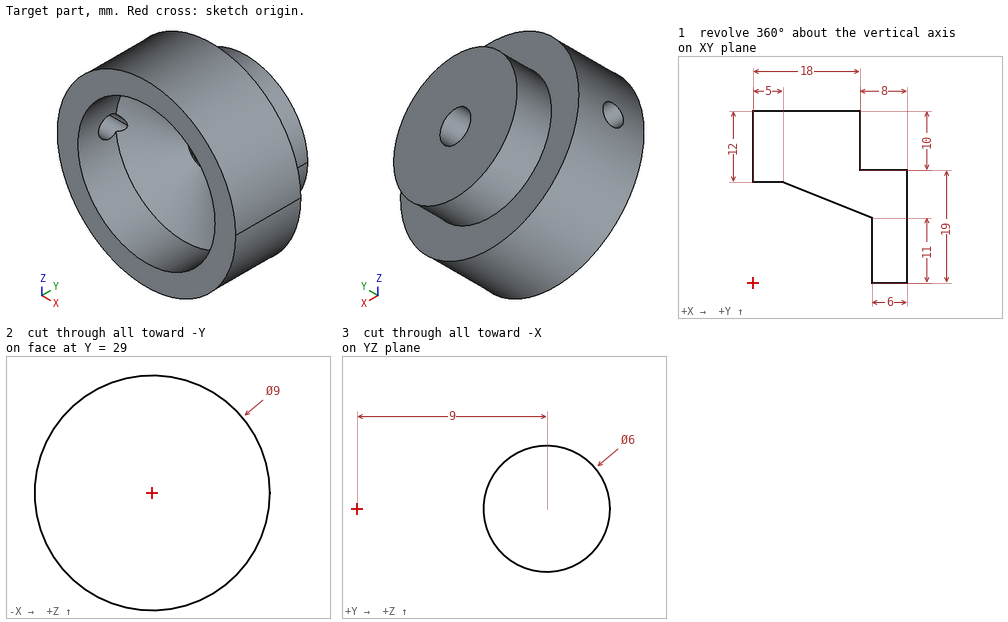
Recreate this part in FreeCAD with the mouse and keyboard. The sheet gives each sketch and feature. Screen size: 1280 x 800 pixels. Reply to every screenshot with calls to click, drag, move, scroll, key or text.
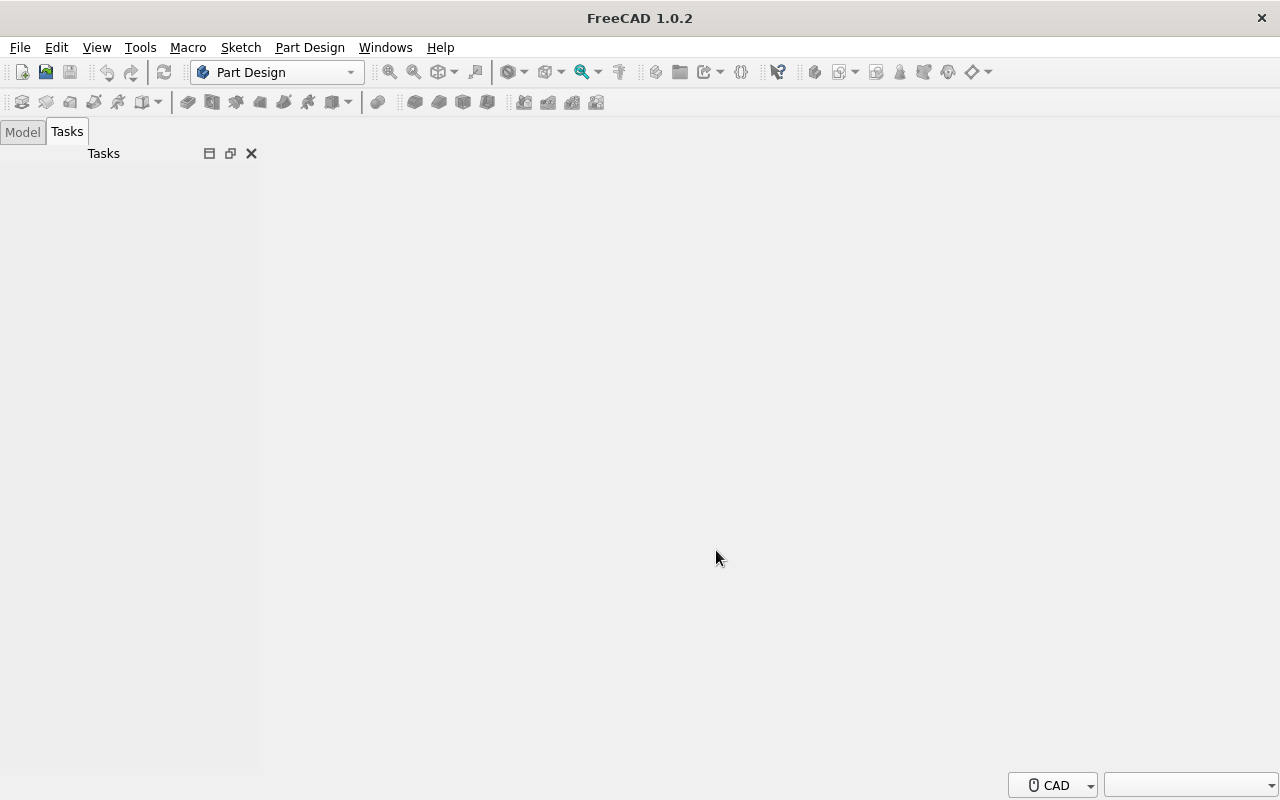
click(22, 72)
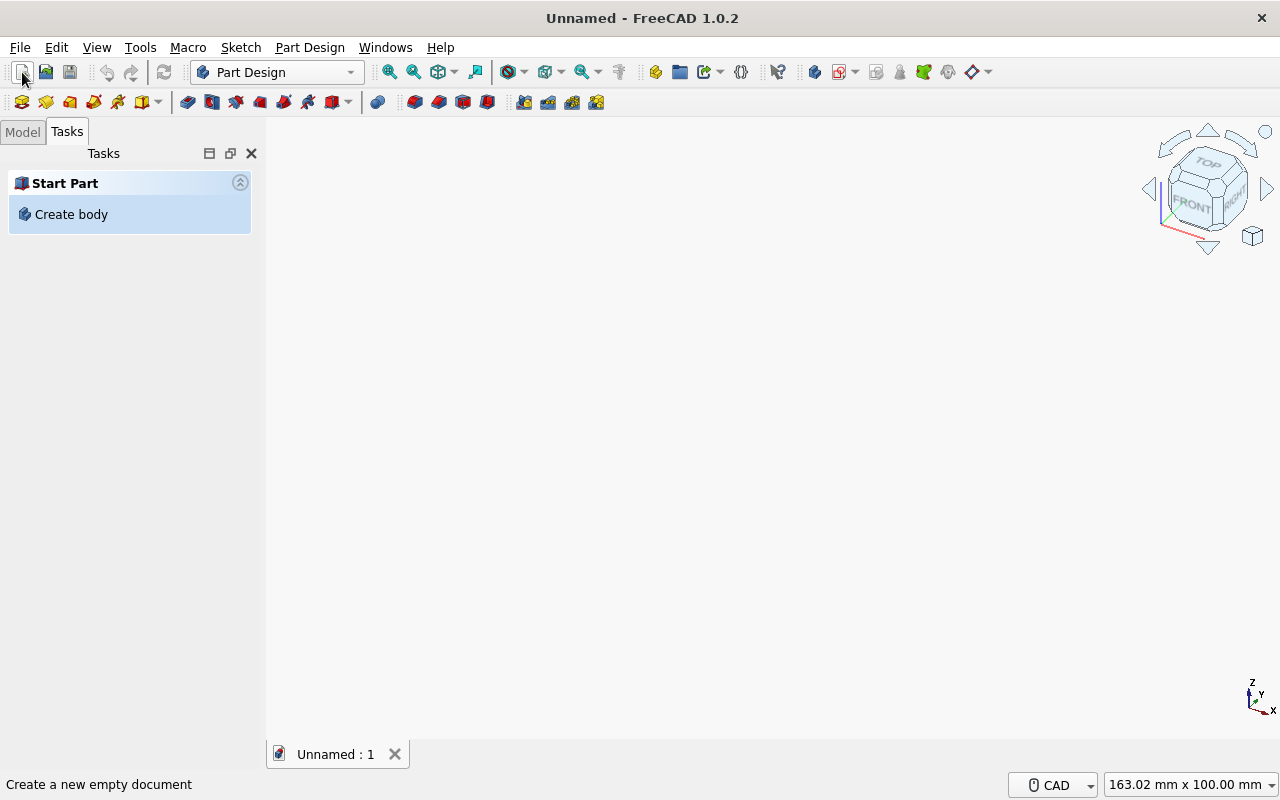
click(840, 72)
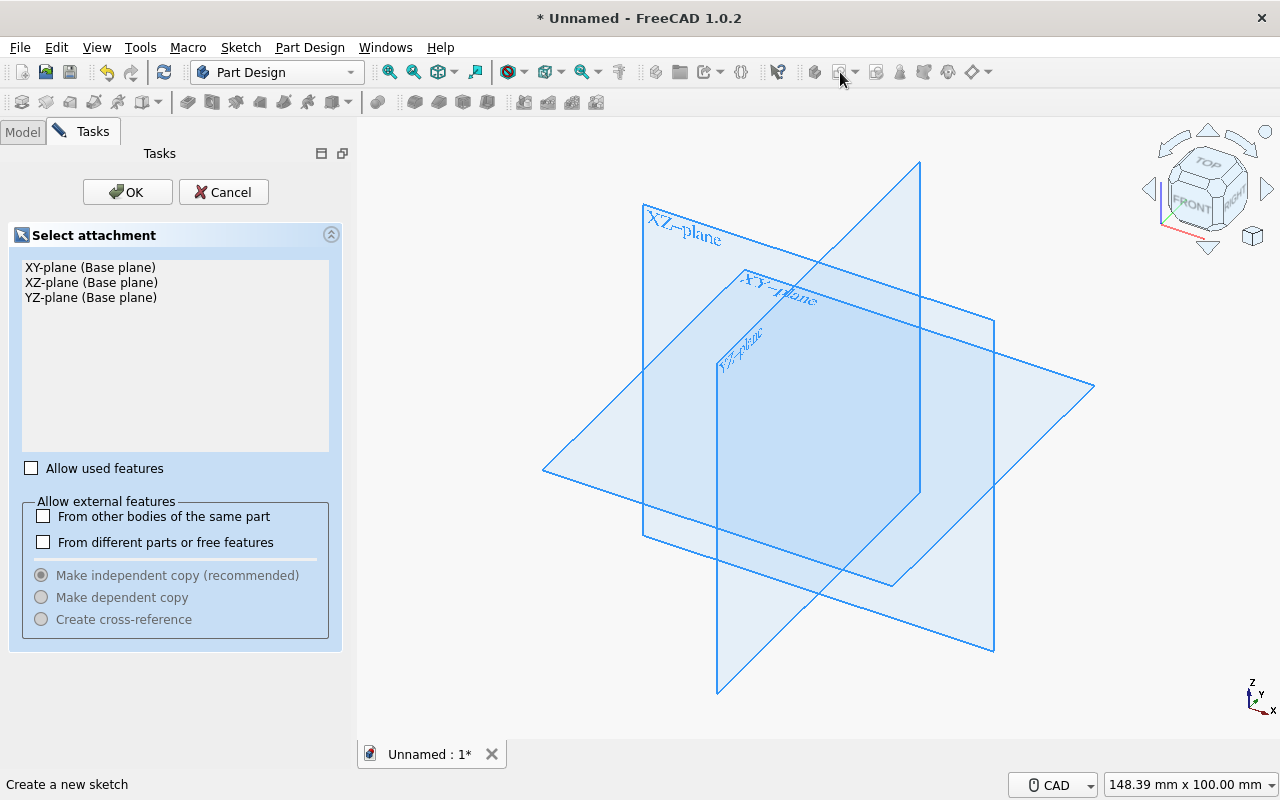
click(82, 268)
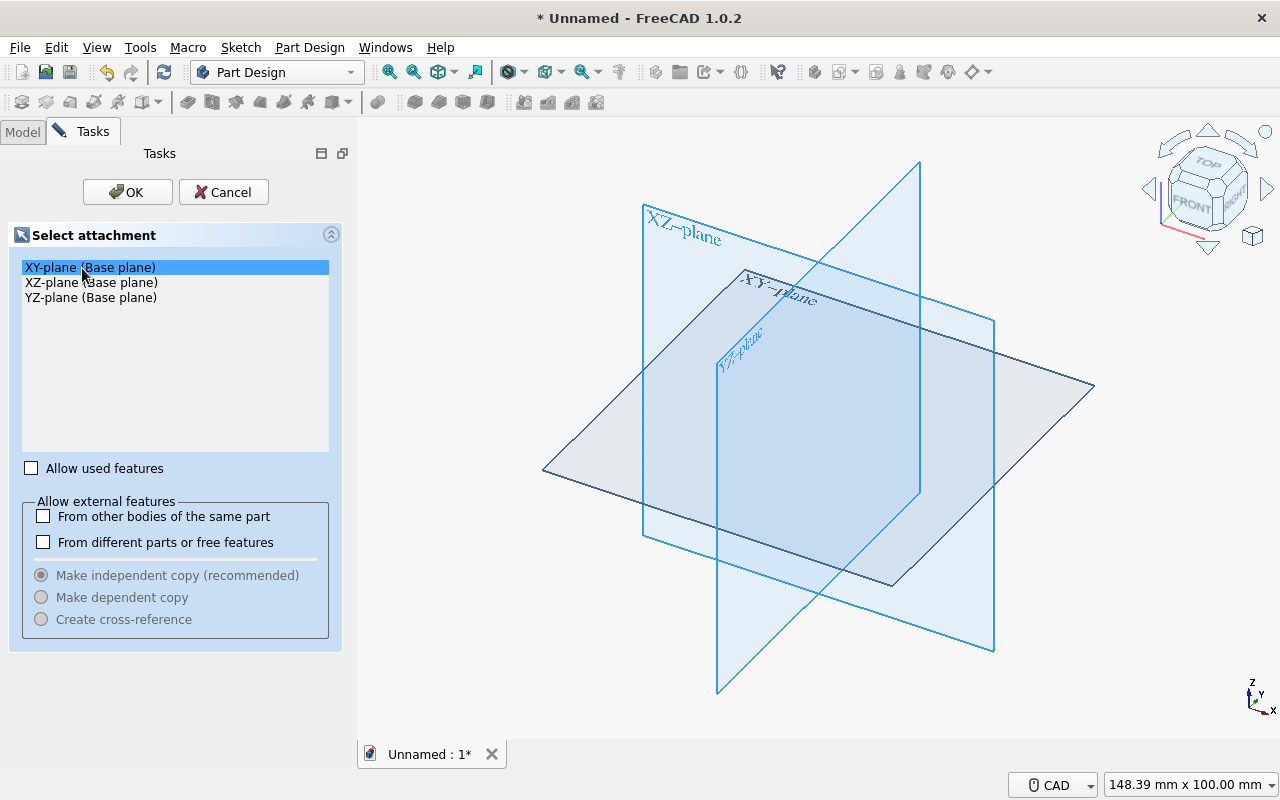
click(128, 192)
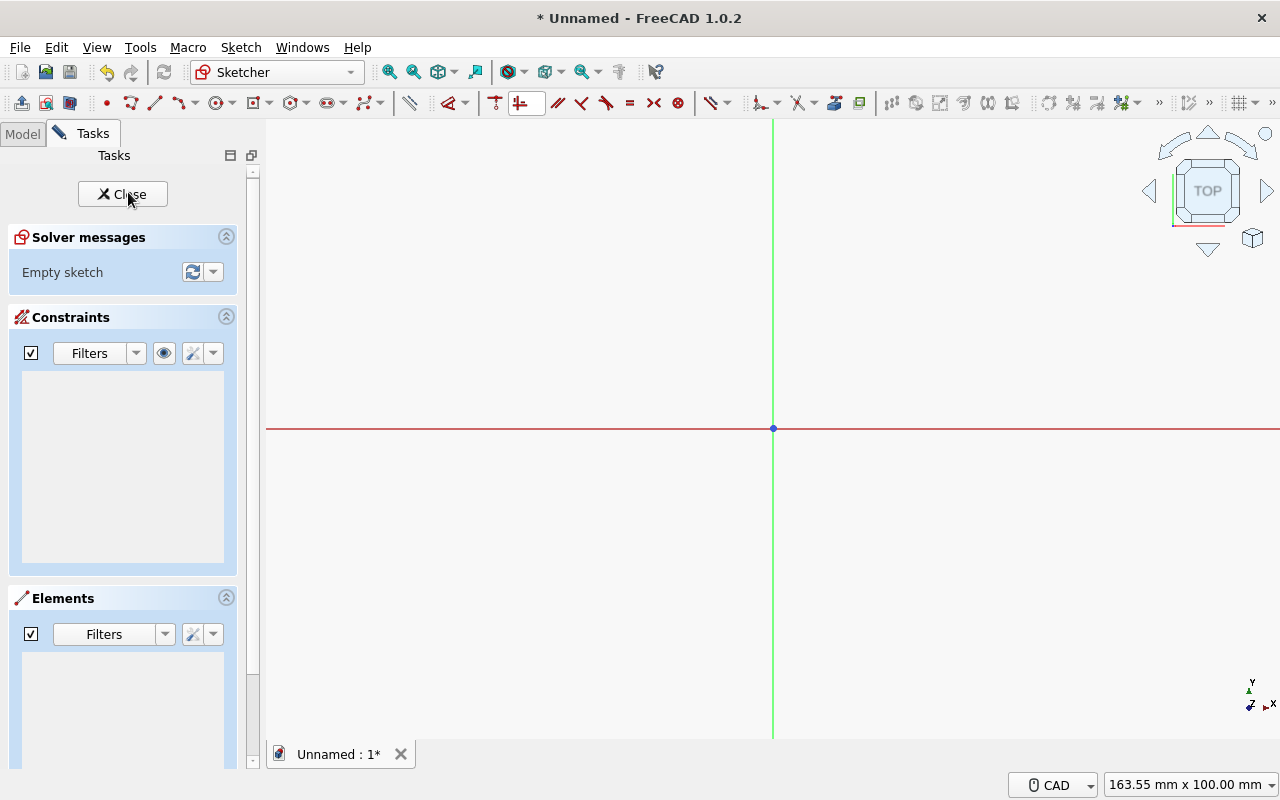
scroll(975, 266, up, 4)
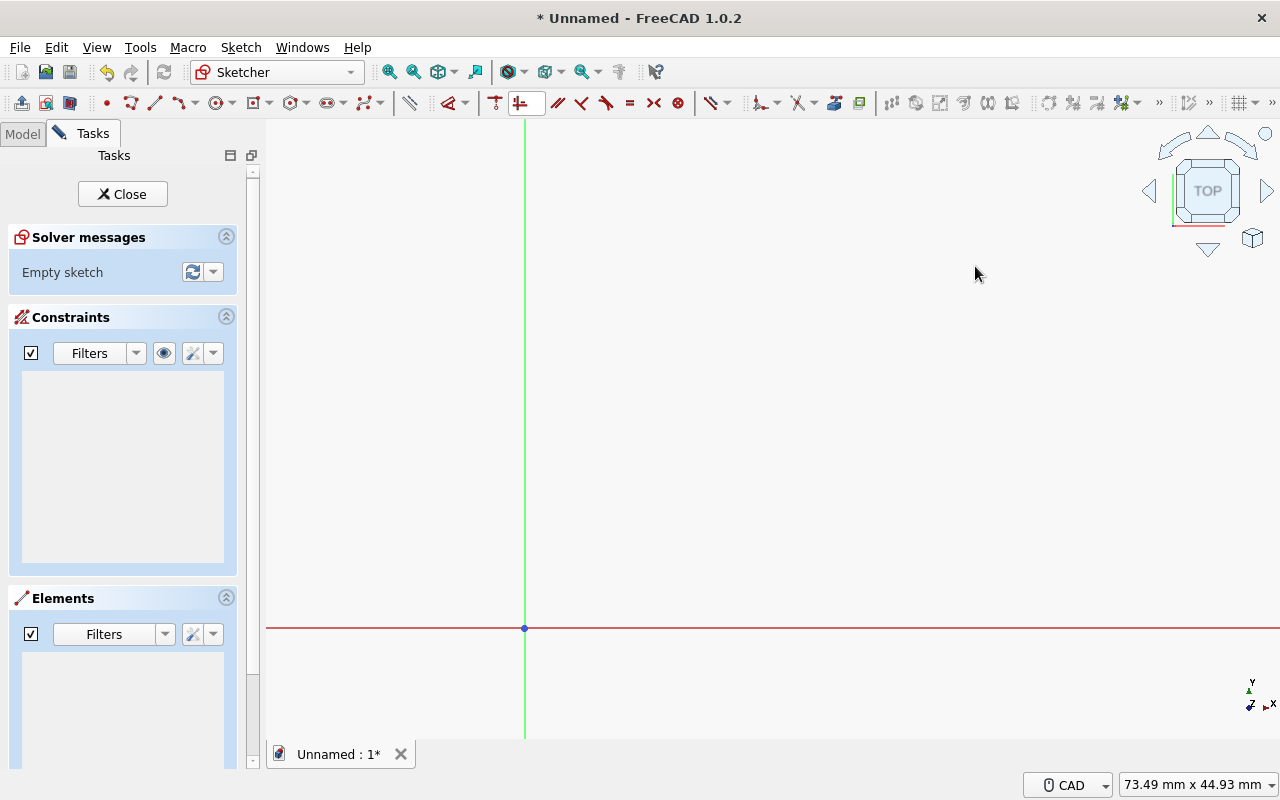
click(132, 104)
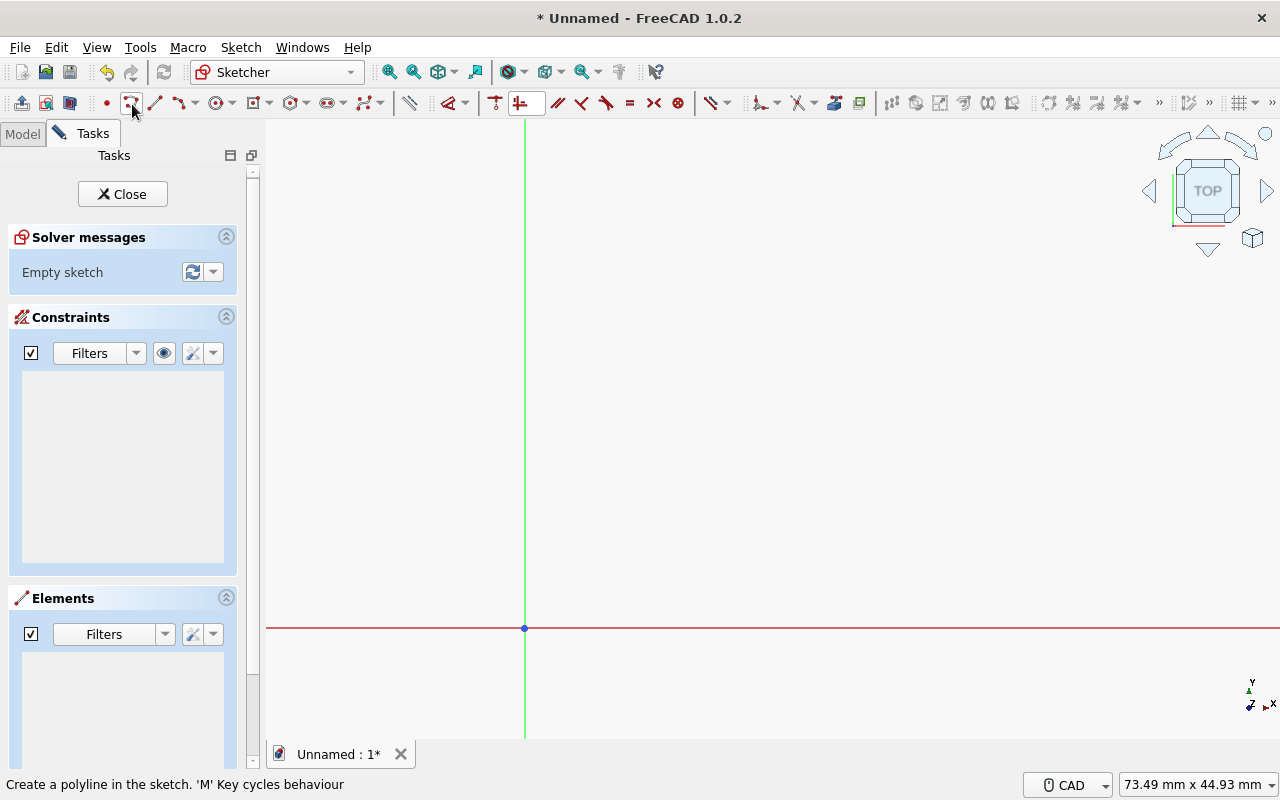
click(525, 394)
click(594, 394)
click(801, 477)
click(801, 628)
click(883, 619)
click(883, 366)
click(773, 366)
click(773, 228)
click(534, 228)
click(525, 395)
key(Escape)
key(Escape)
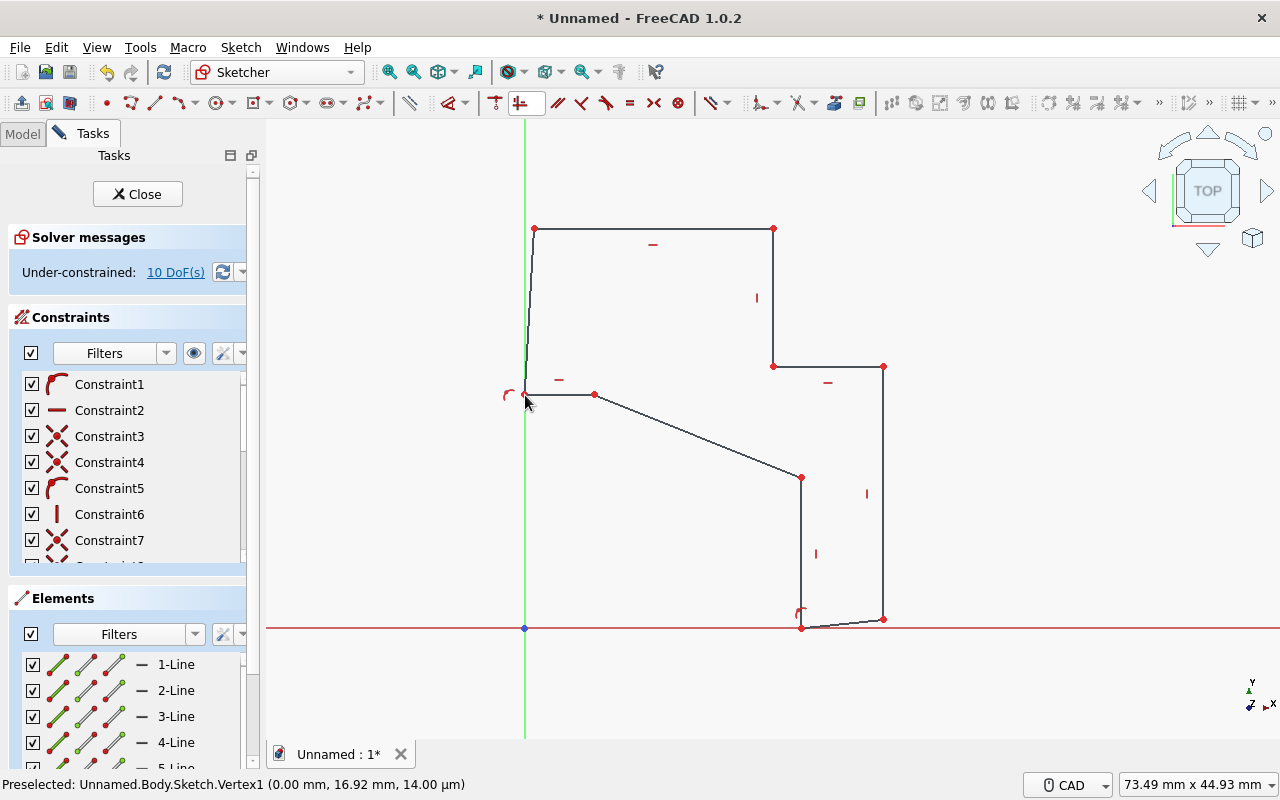
click(826, 626)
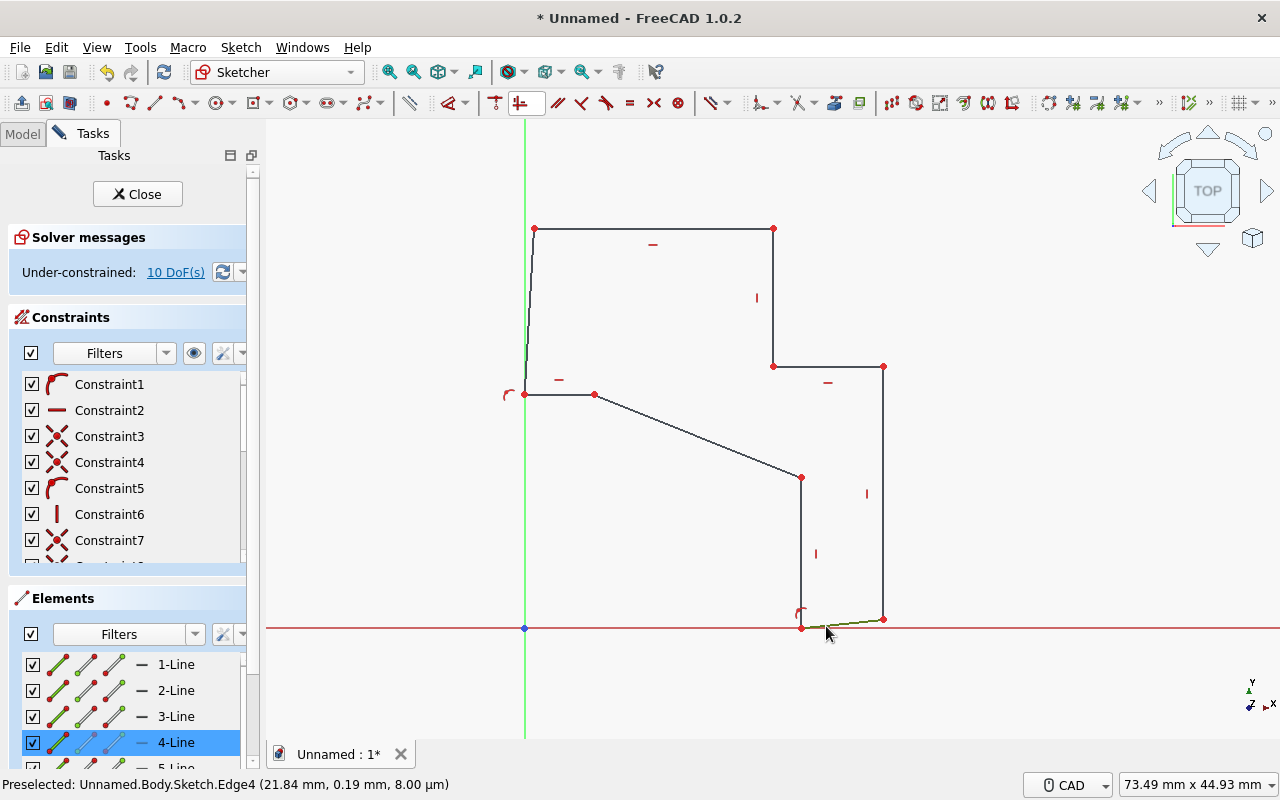
click(540, 104)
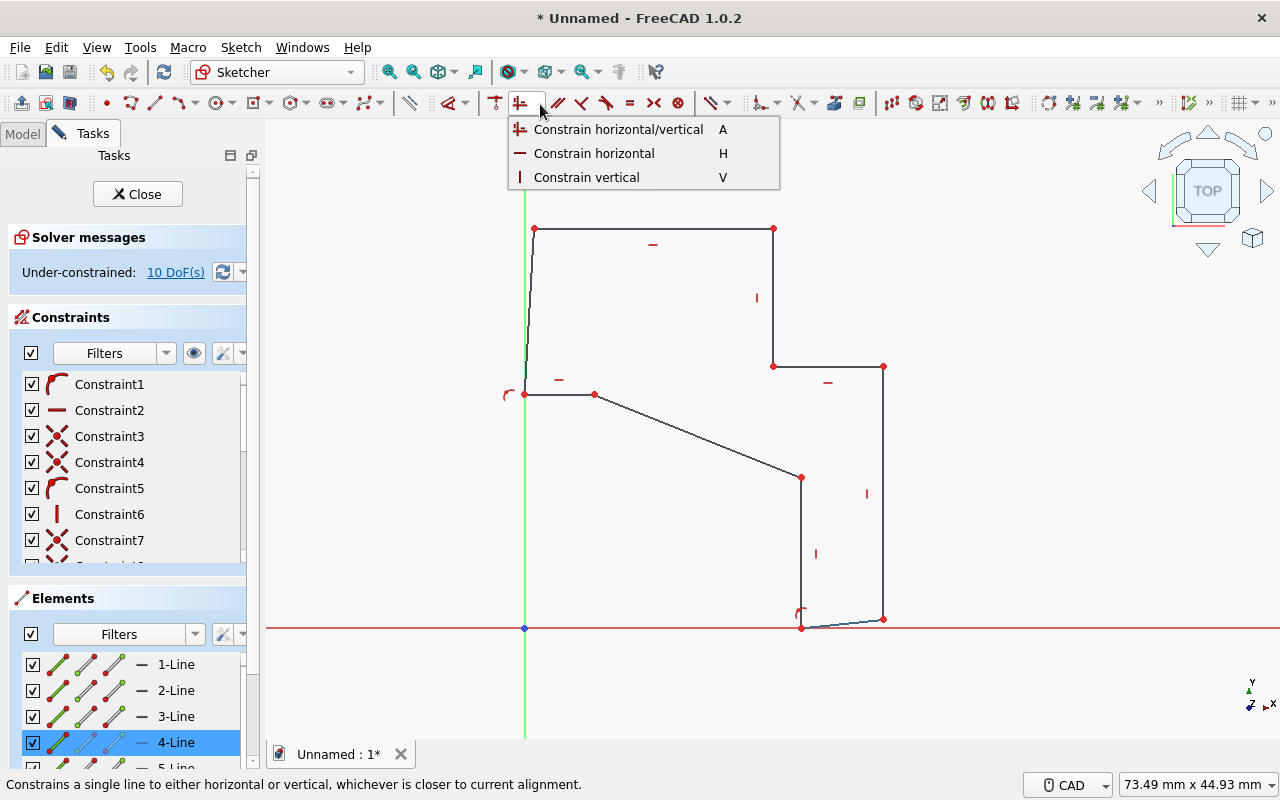
click(644, 153)